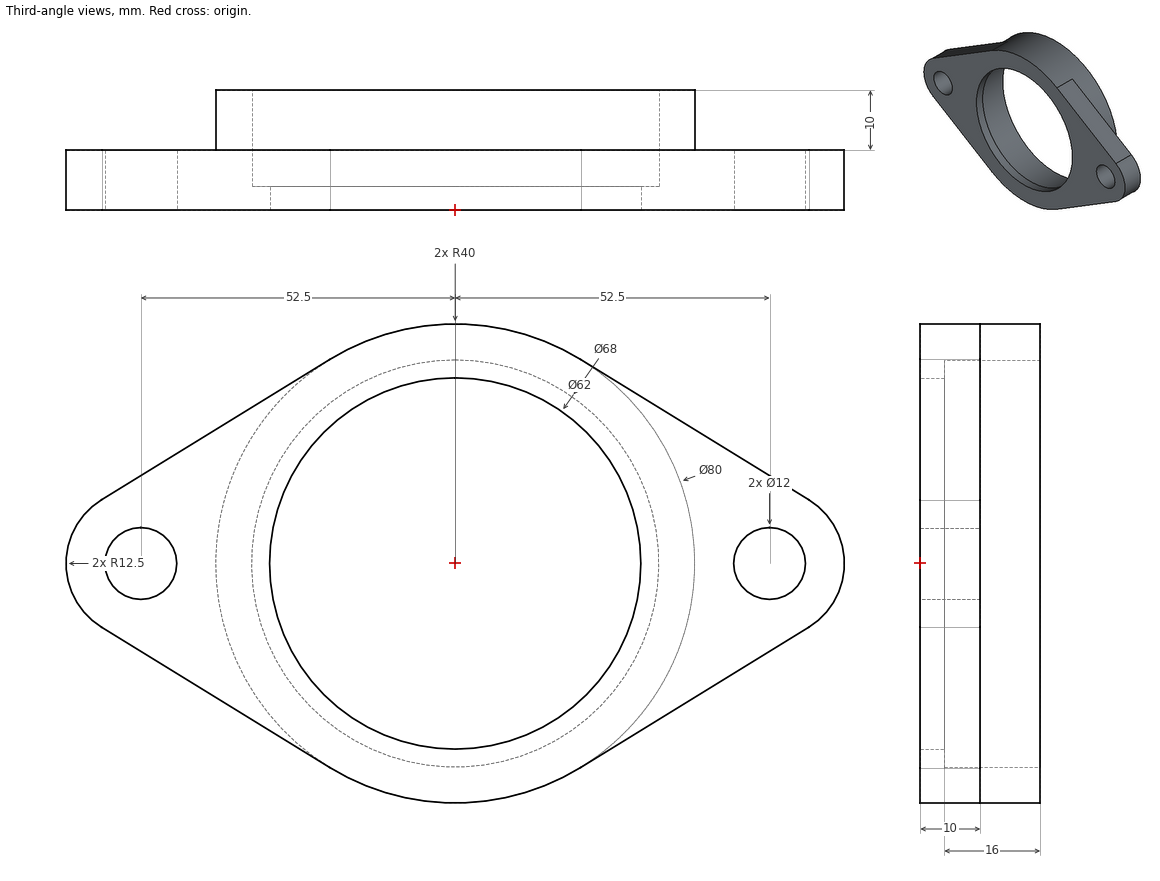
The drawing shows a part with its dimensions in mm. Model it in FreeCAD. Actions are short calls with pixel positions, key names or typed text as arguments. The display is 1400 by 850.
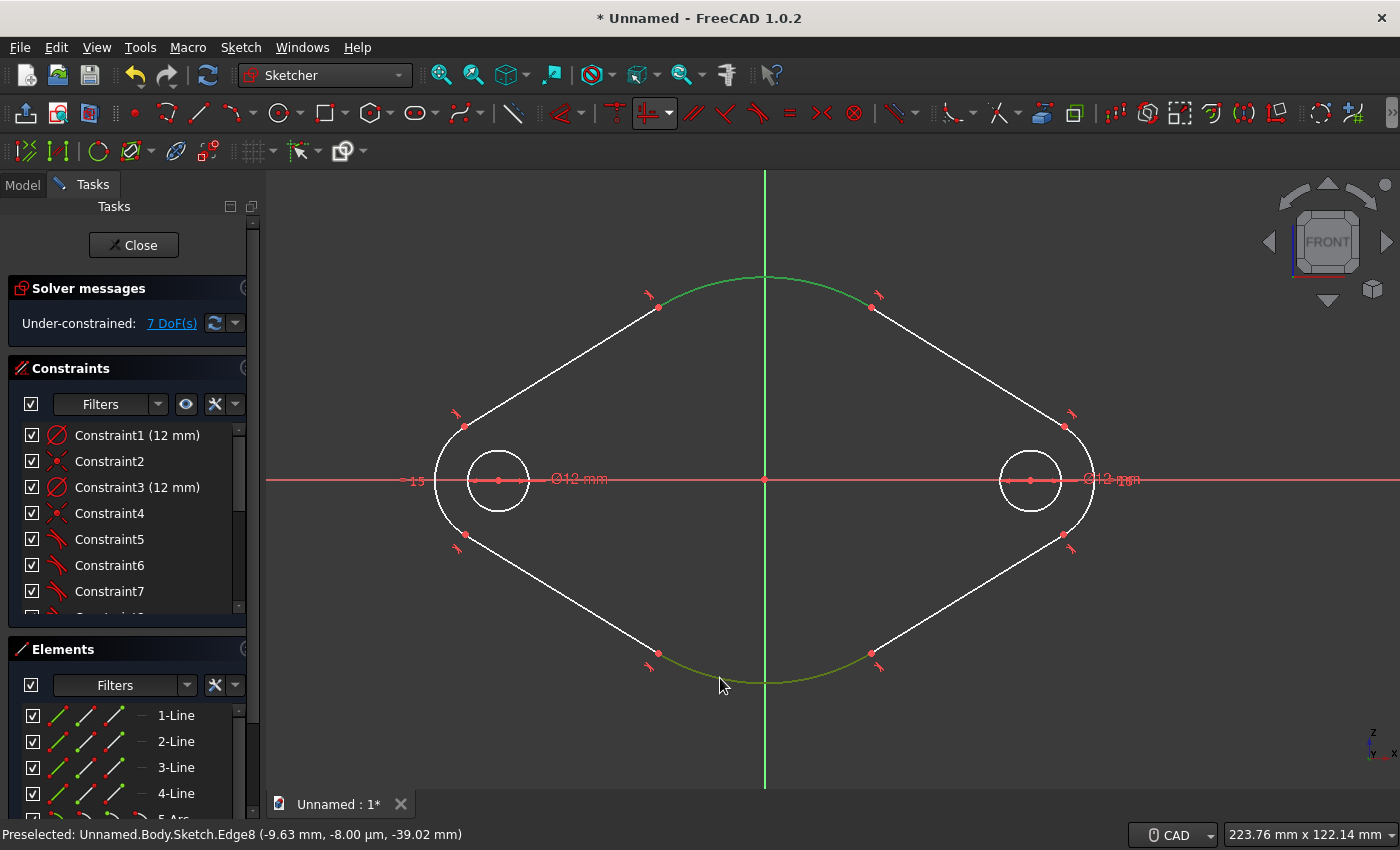
click(790, 114)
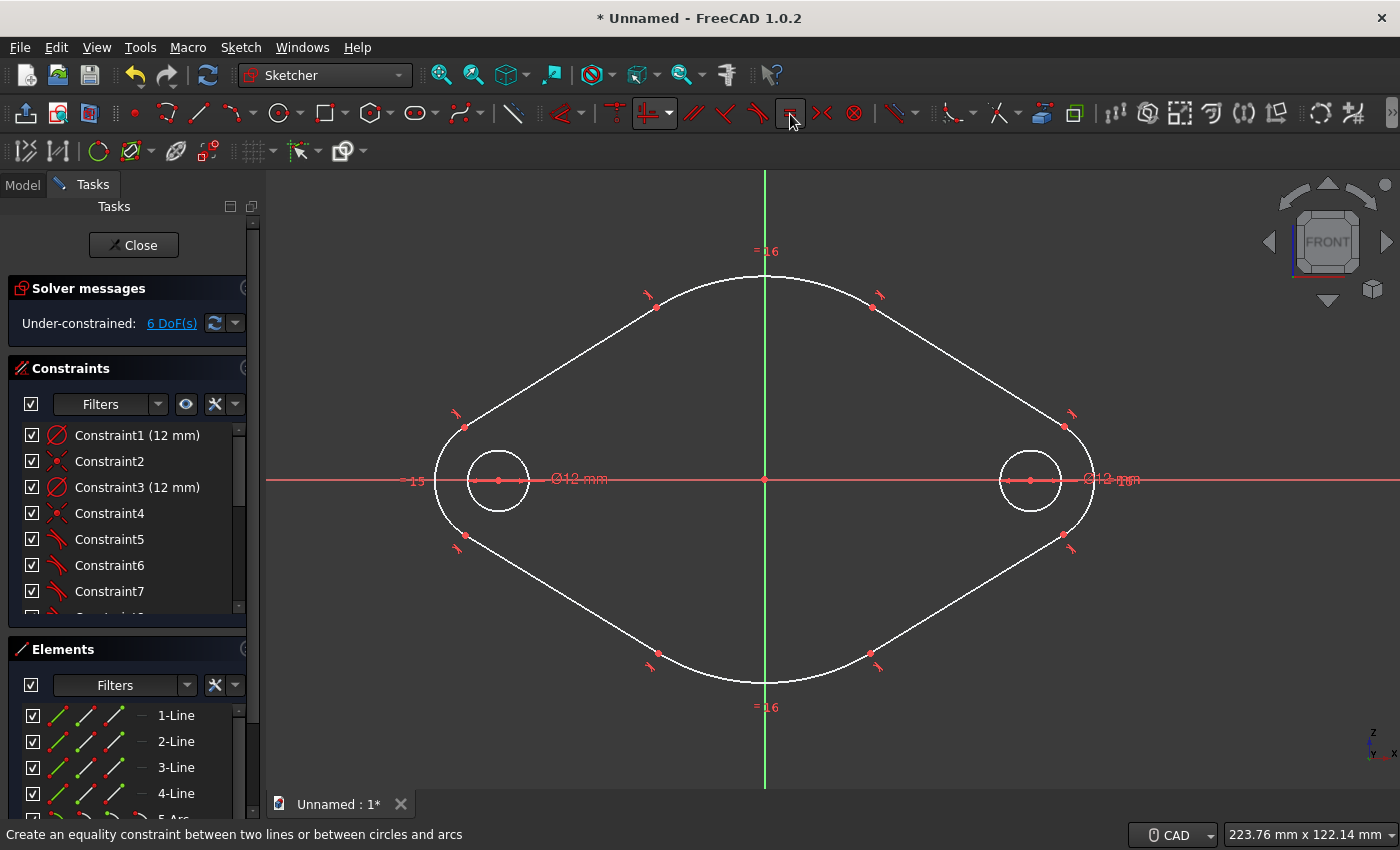
click(498, 481)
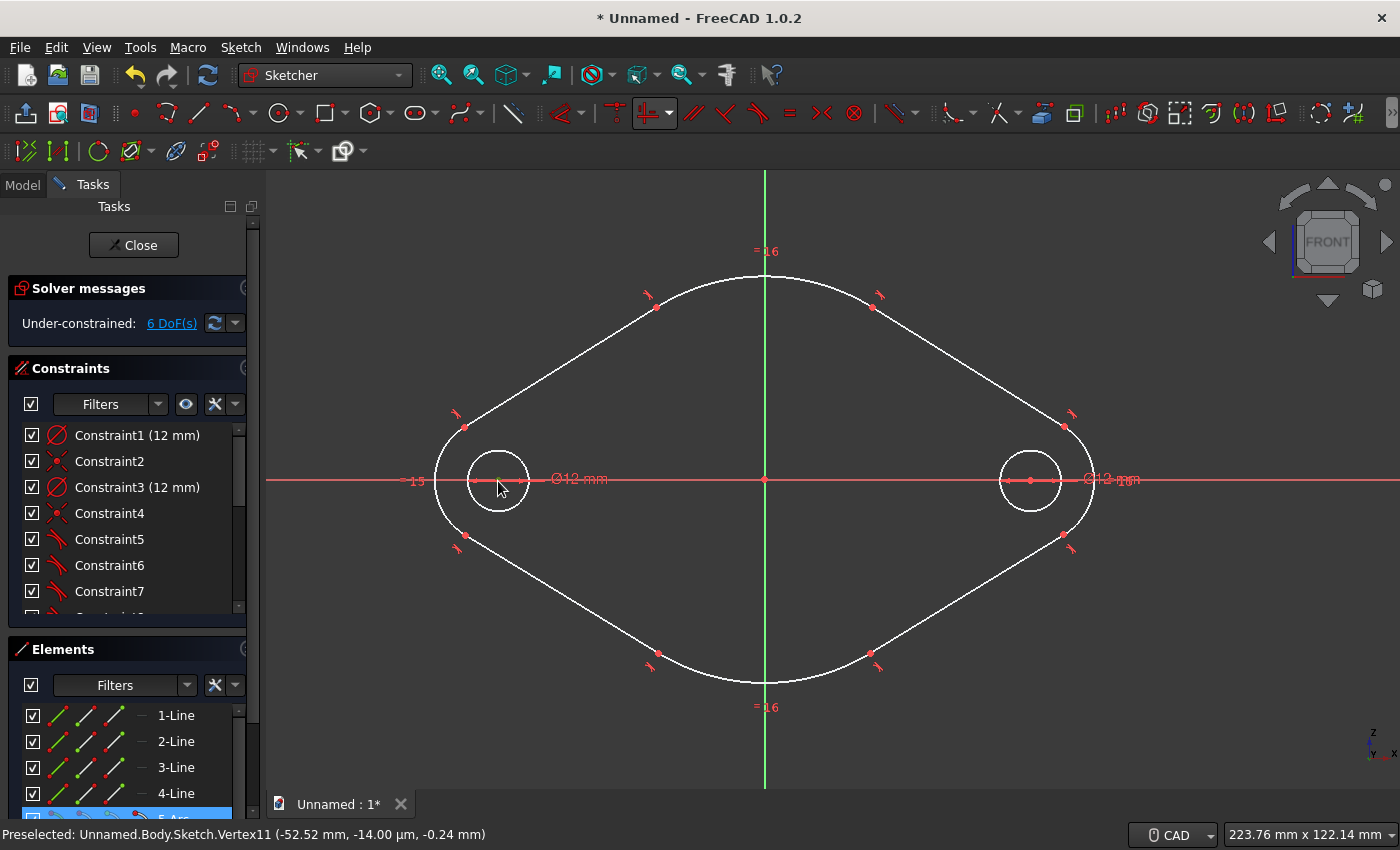
click(361, 480)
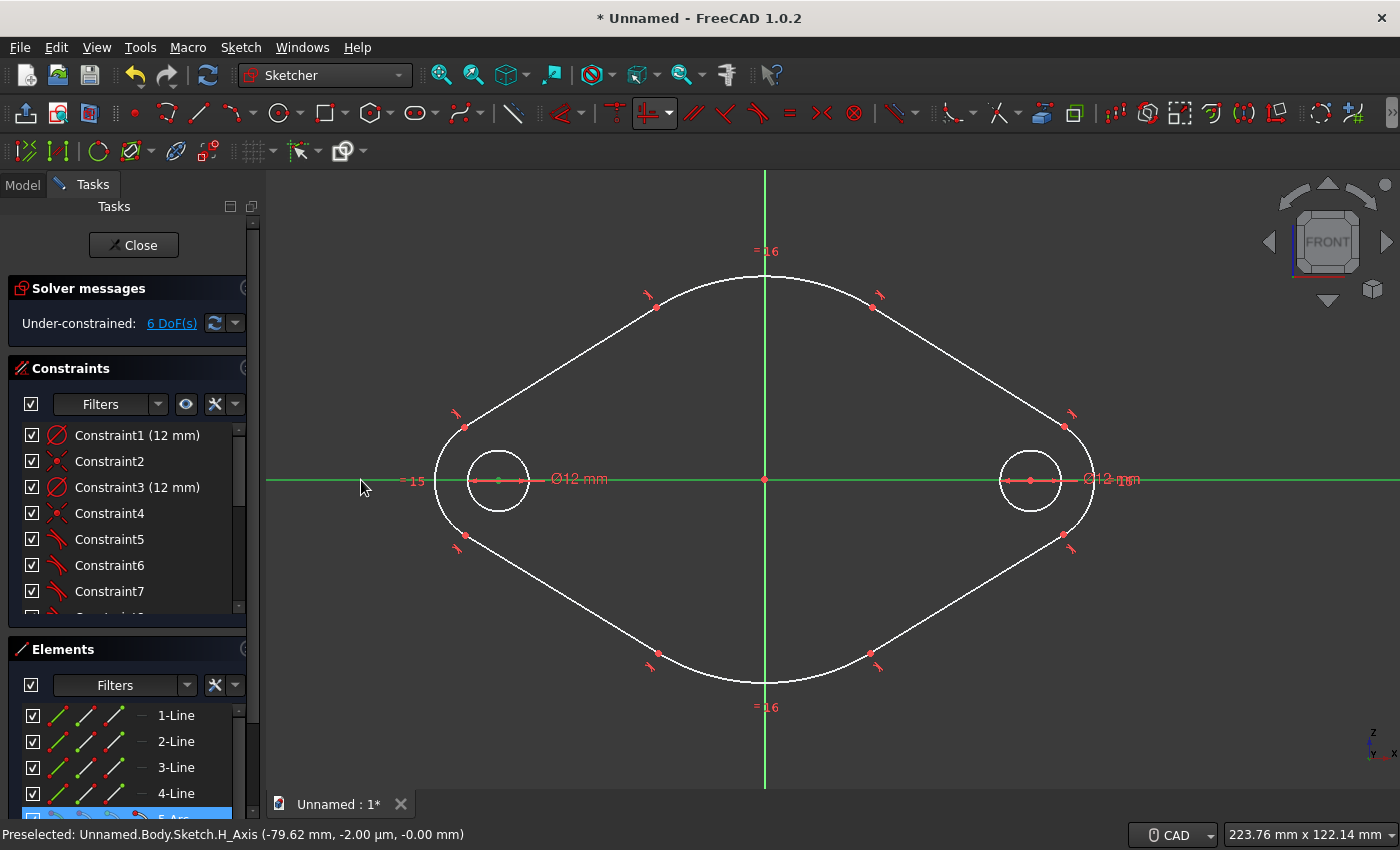
click(616, 114)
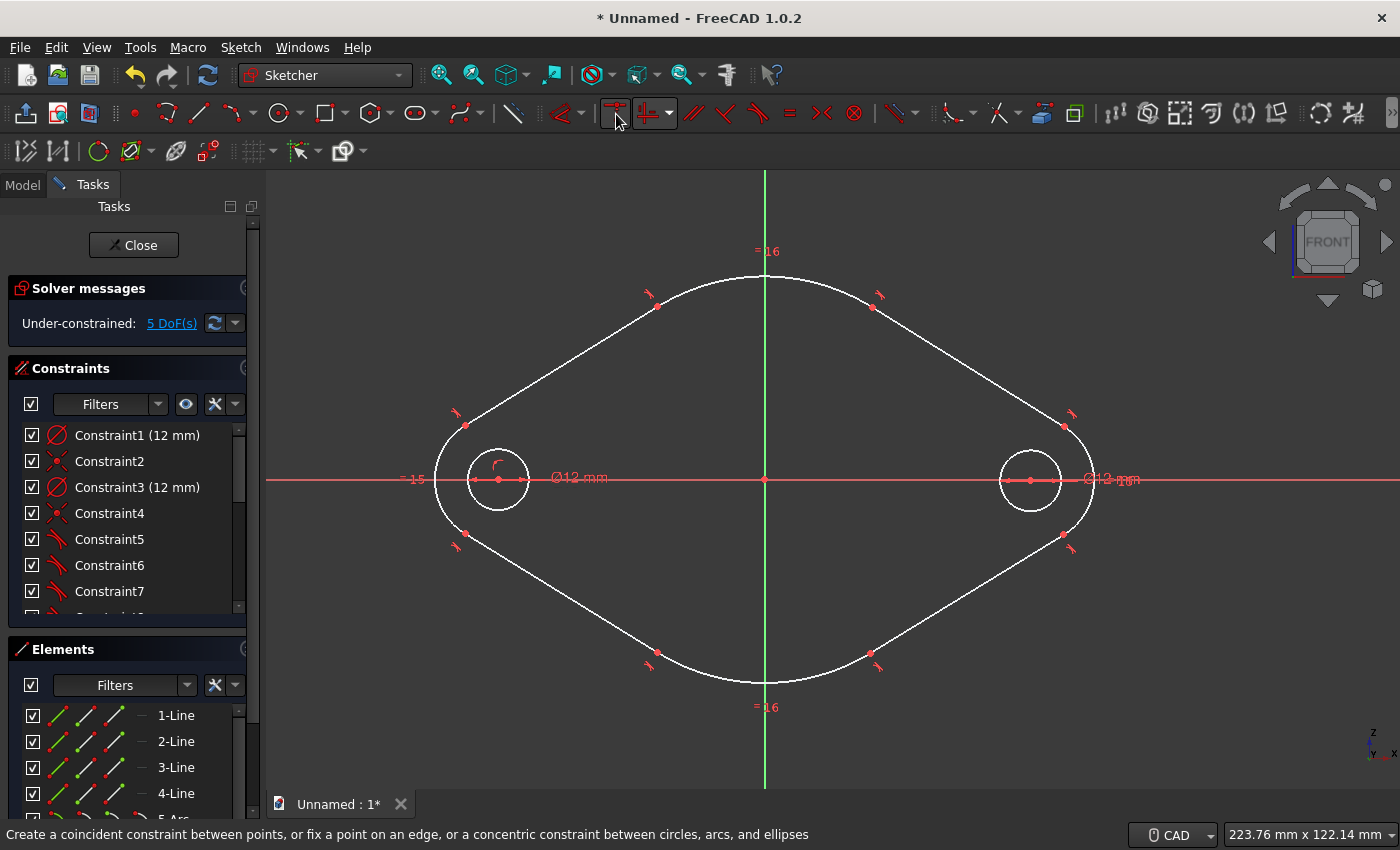
click(1031, 481)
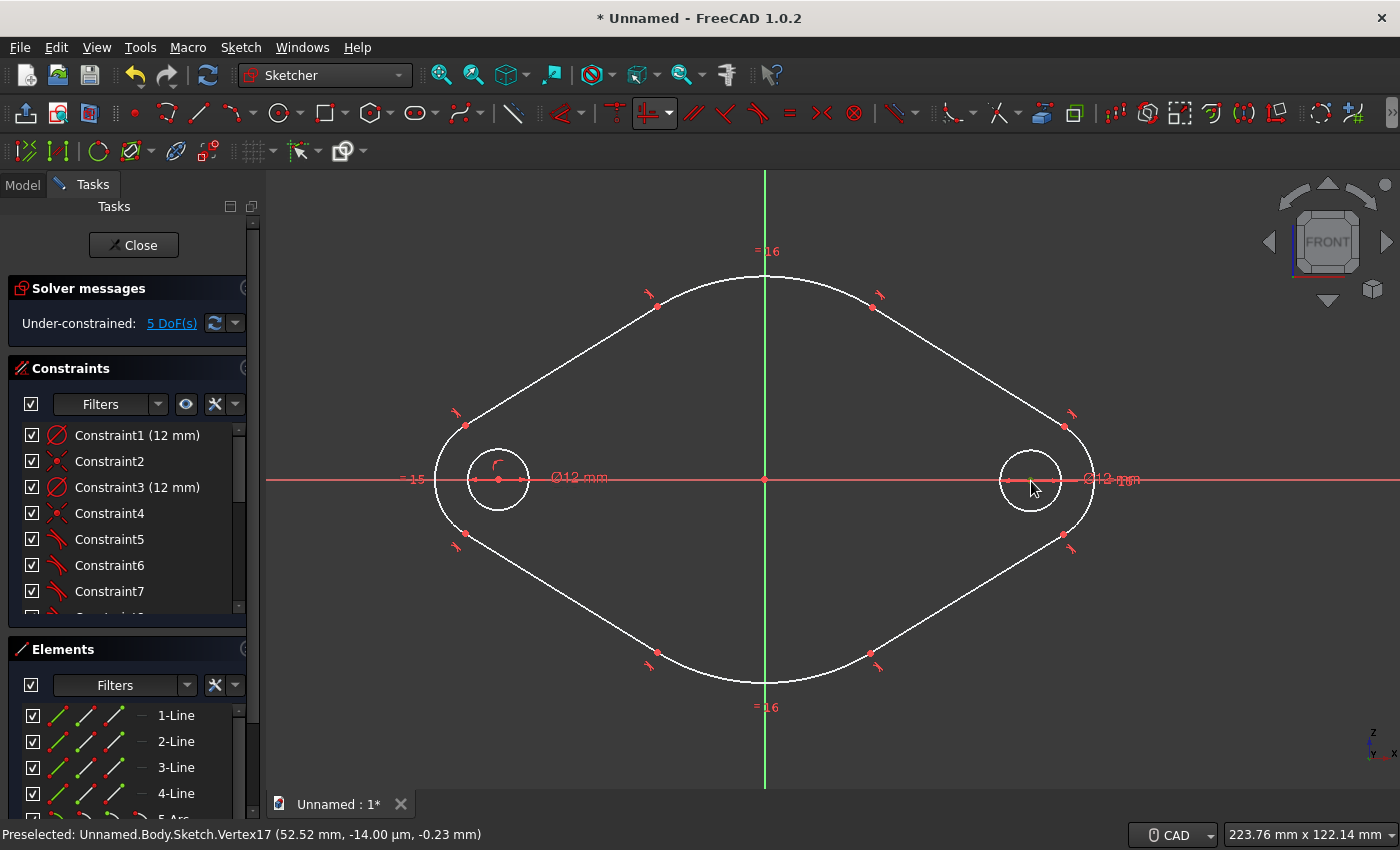
click(361, 480)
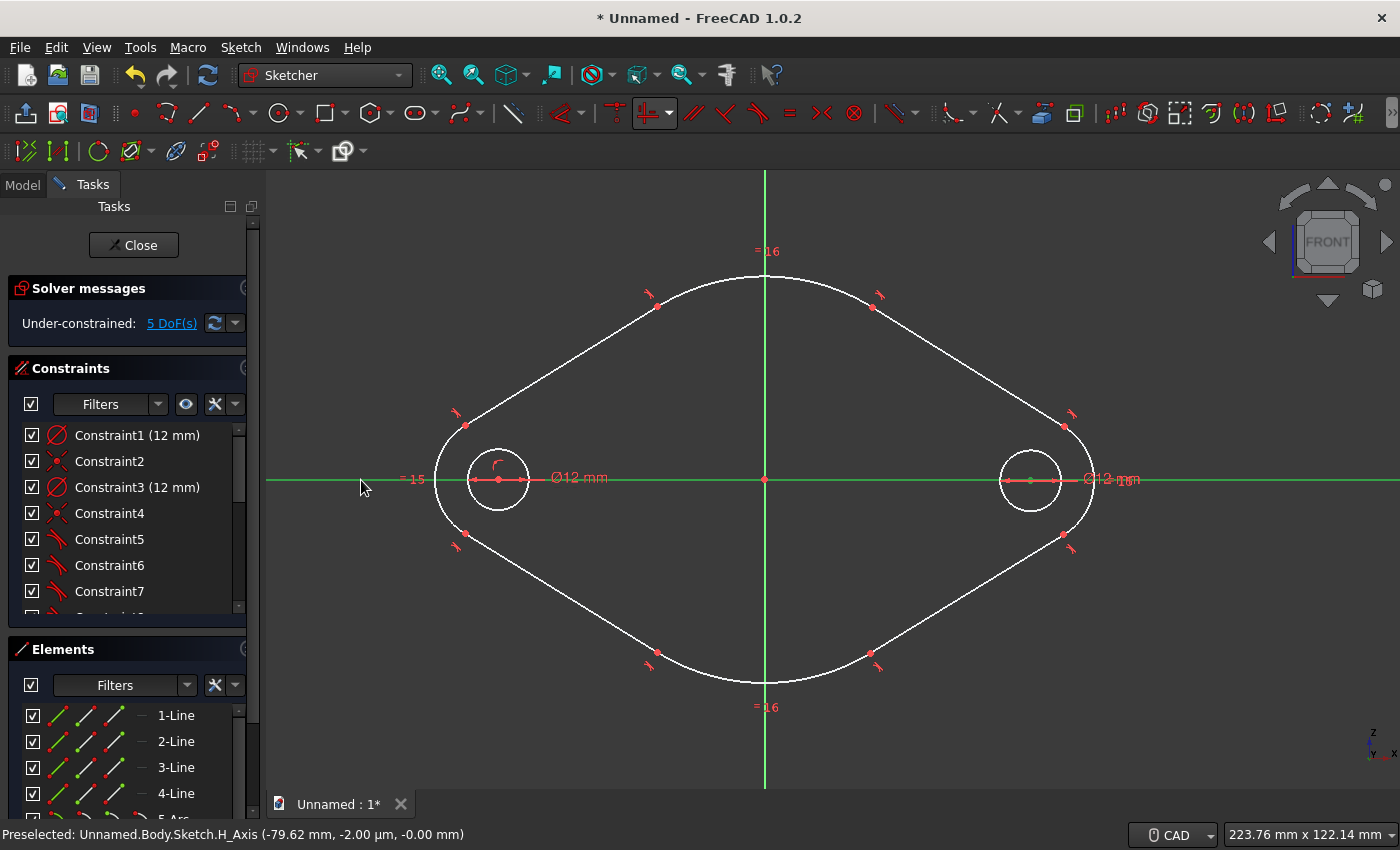
click(616, 114)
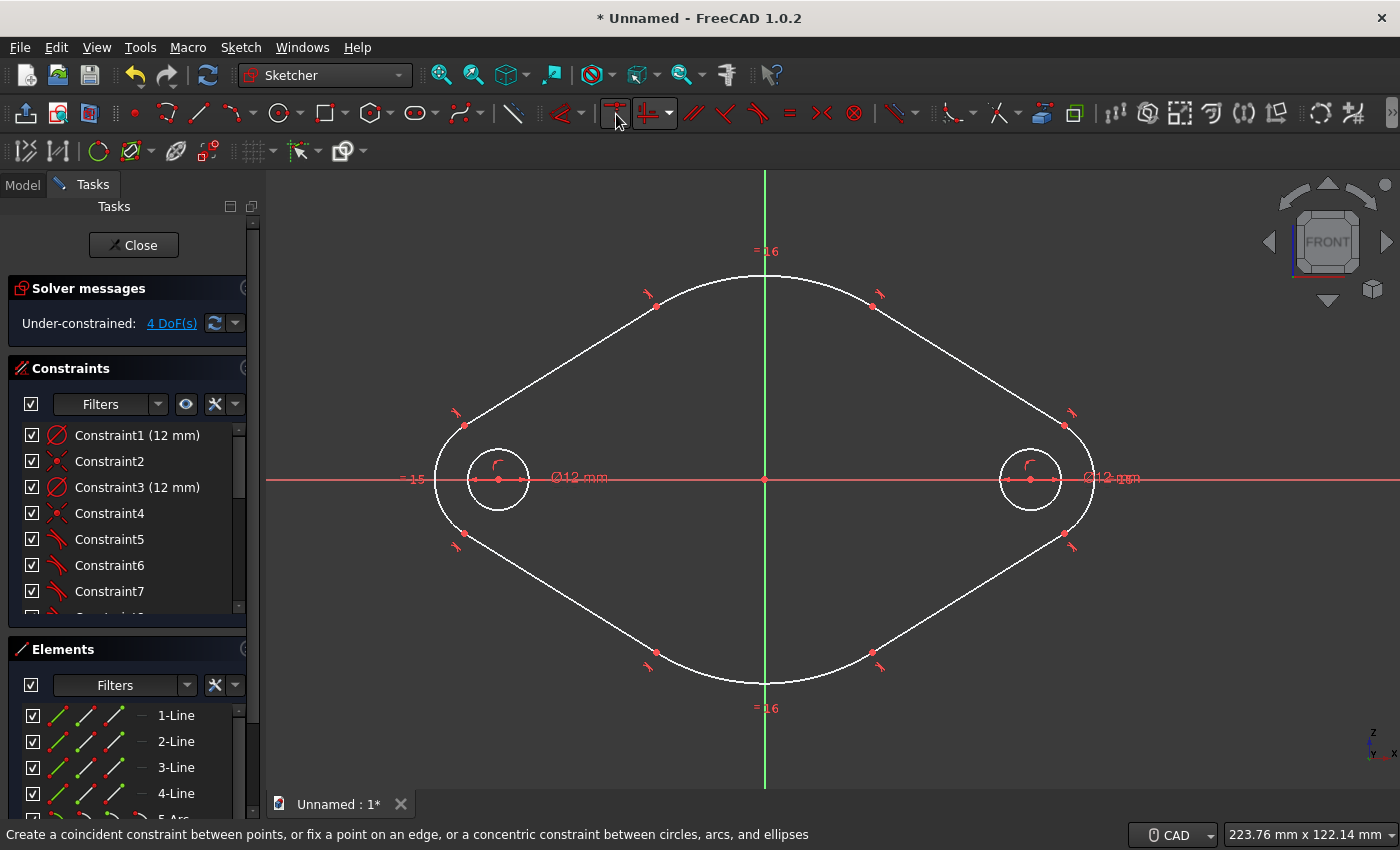
click(560, 114)